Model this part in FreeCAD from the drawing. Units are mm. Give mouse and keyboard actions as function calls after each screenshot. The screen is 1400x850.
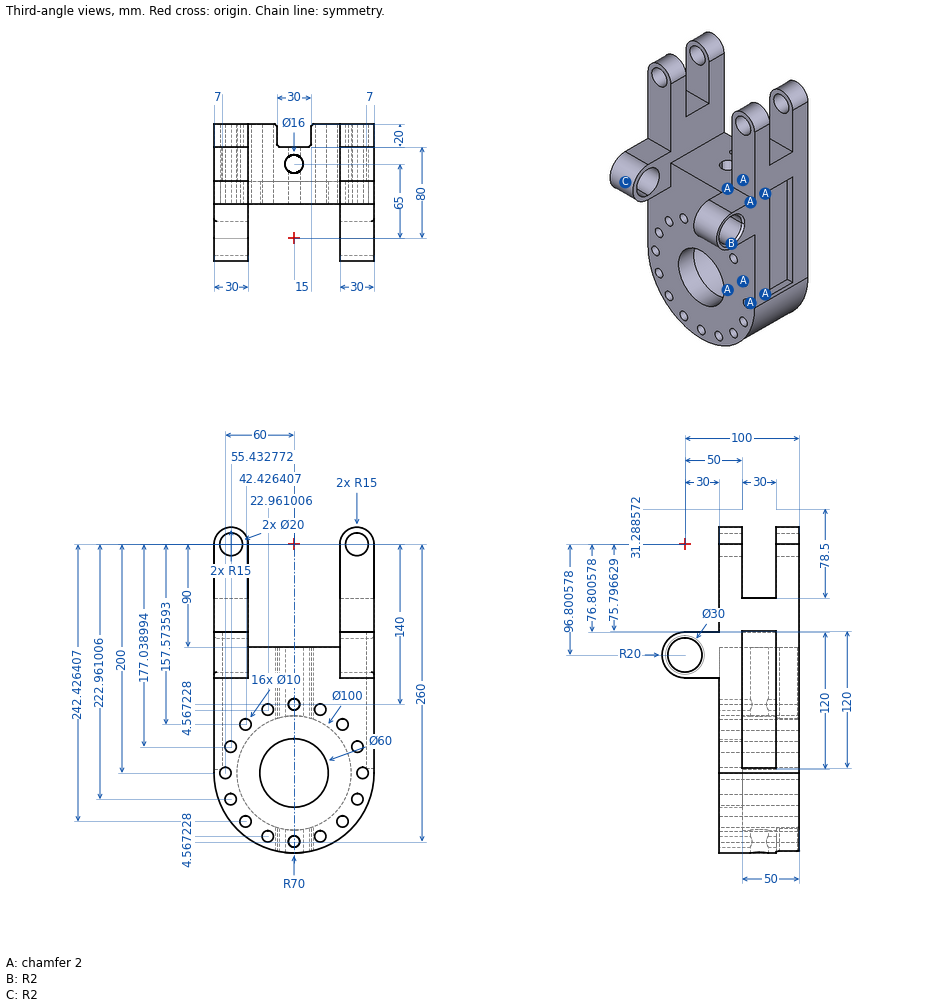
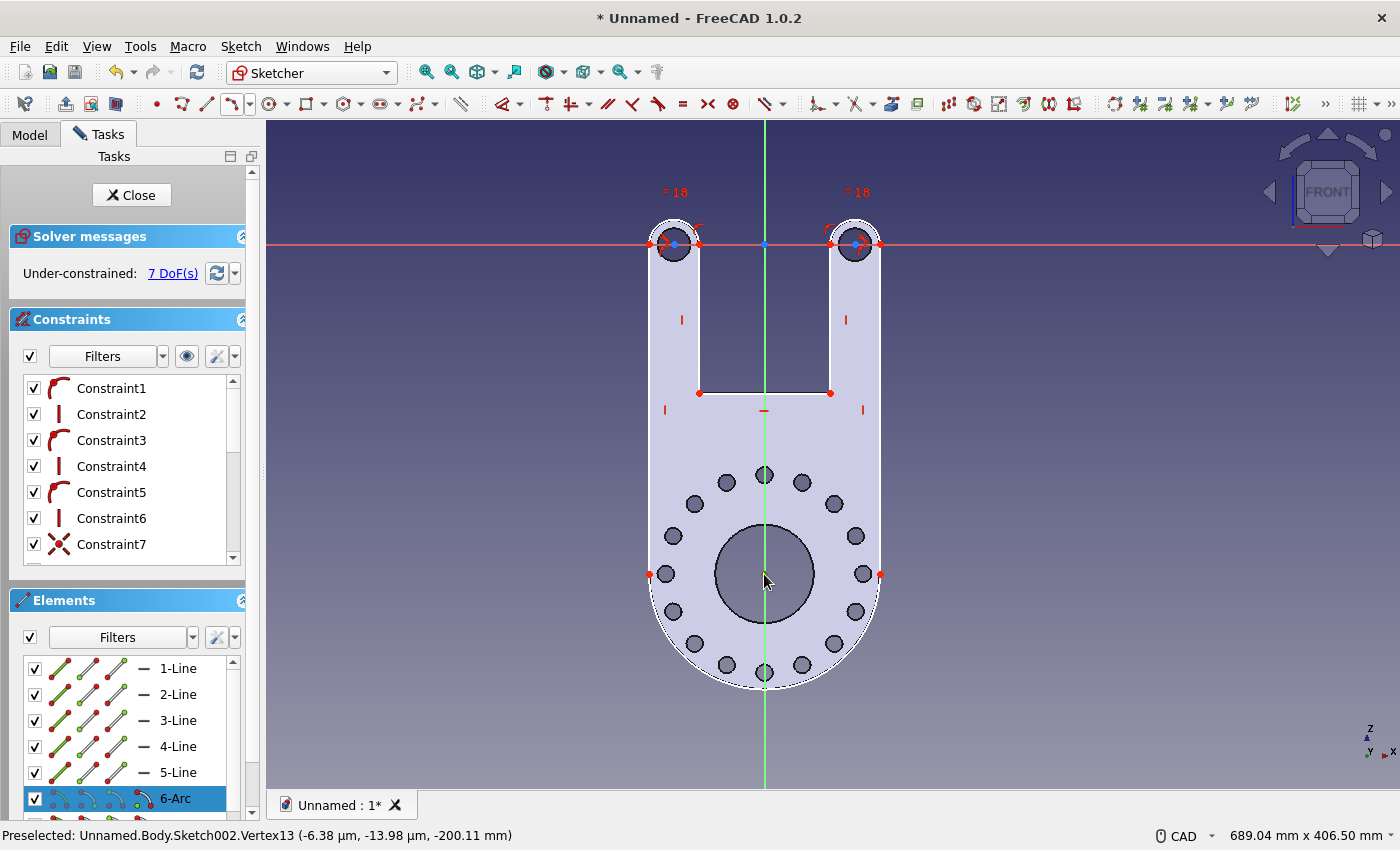
click(765, 630)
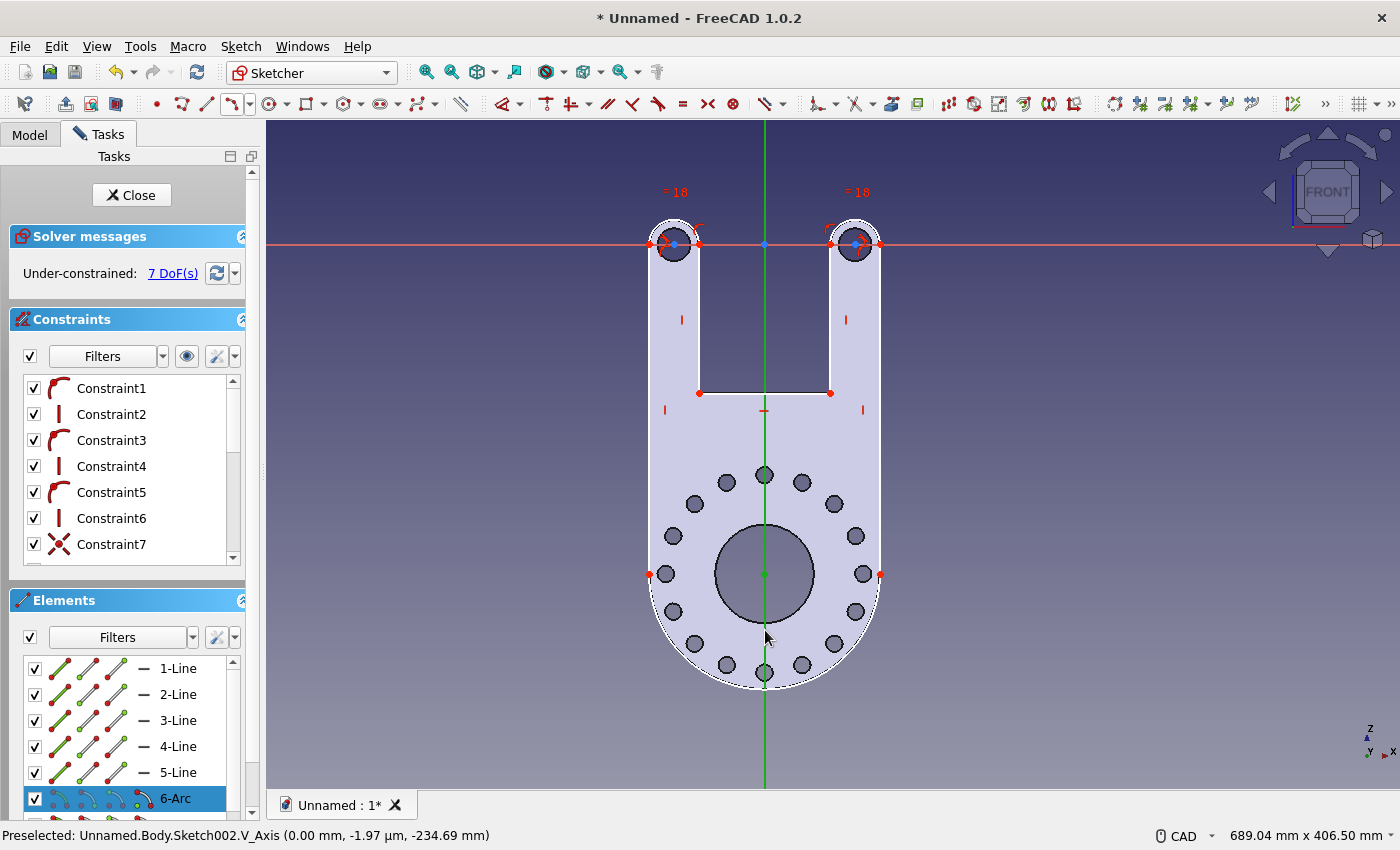
key(c)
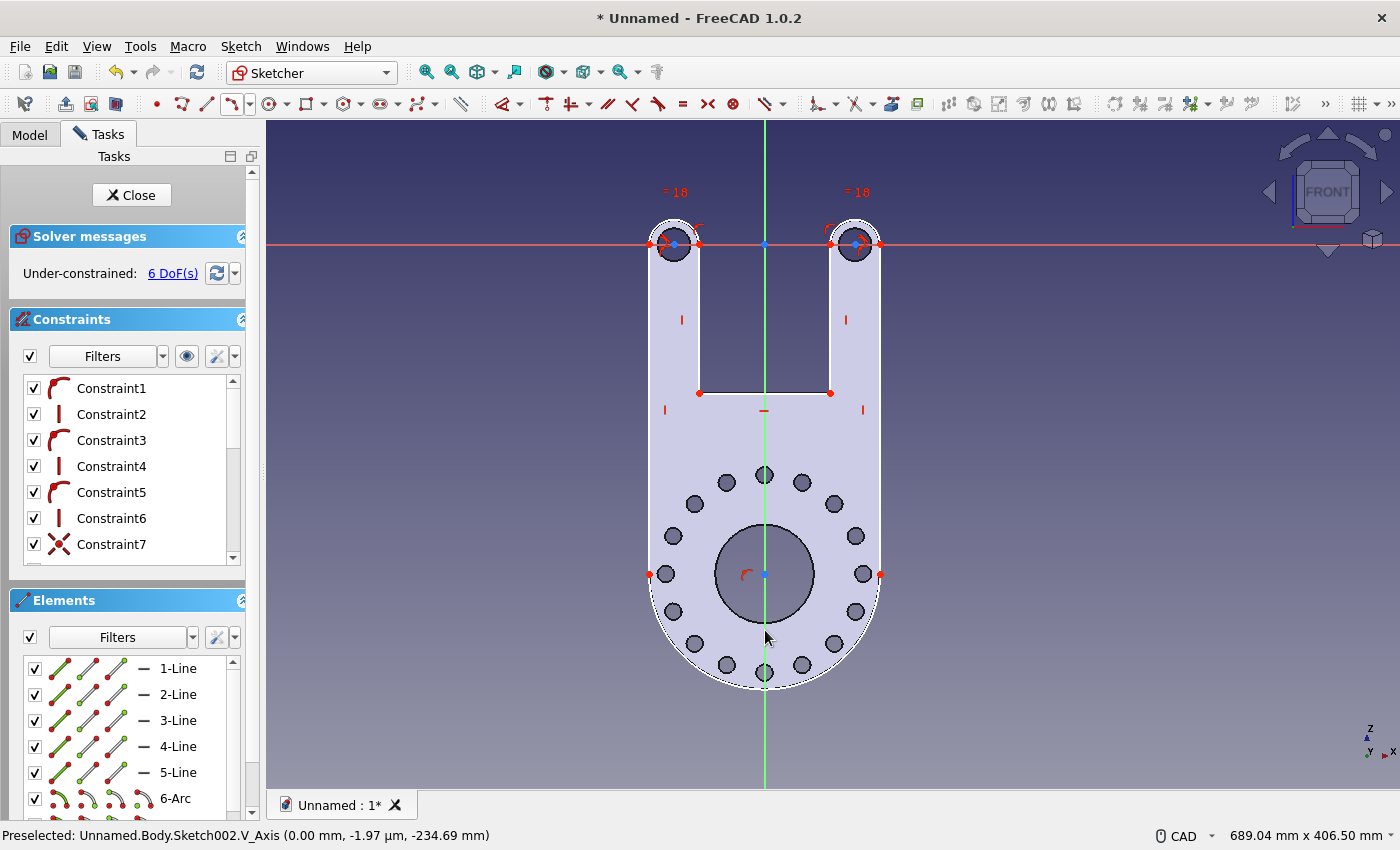
key(d)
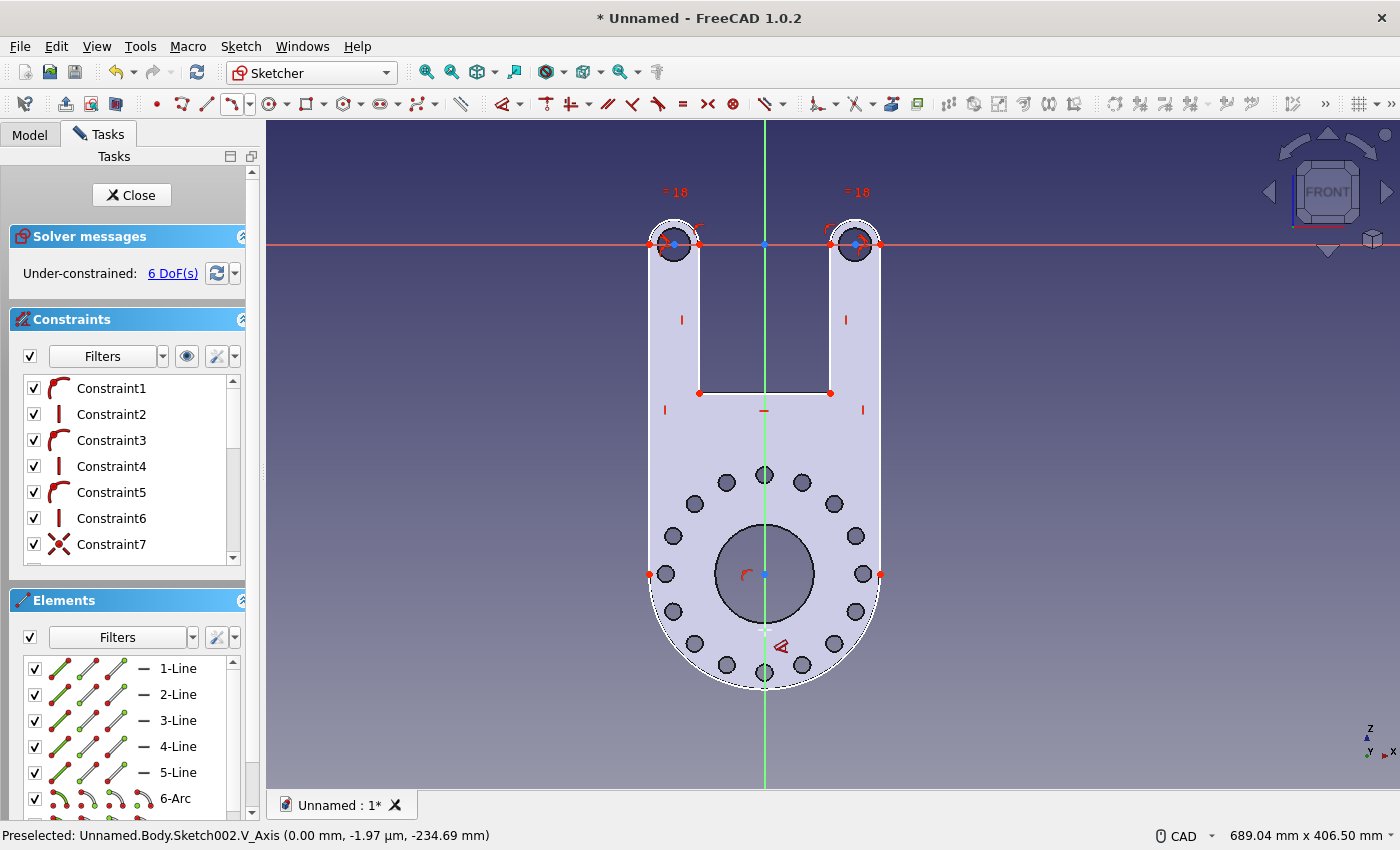
click(697, 668)
click(678, 694)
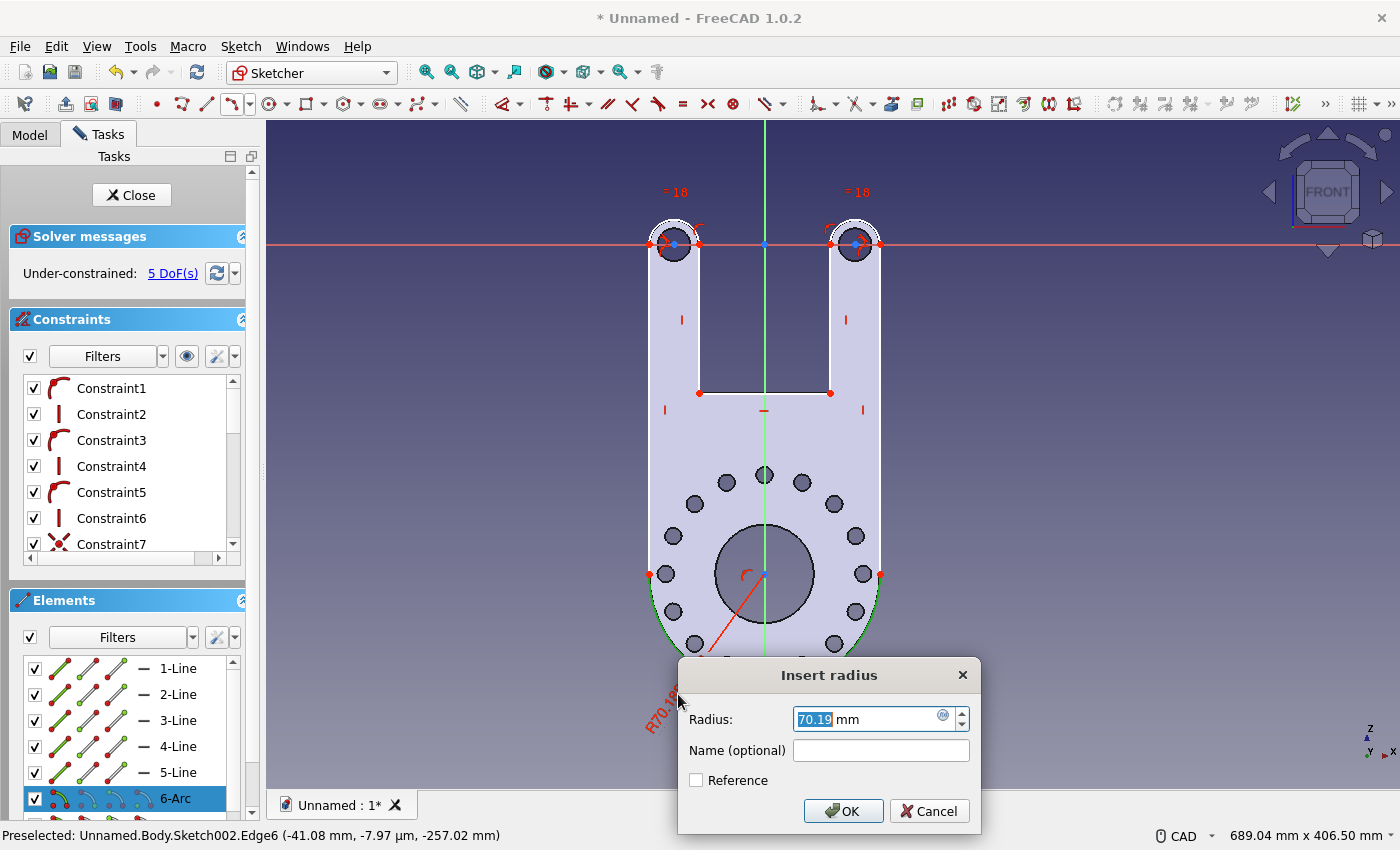
text(70)
key(Return)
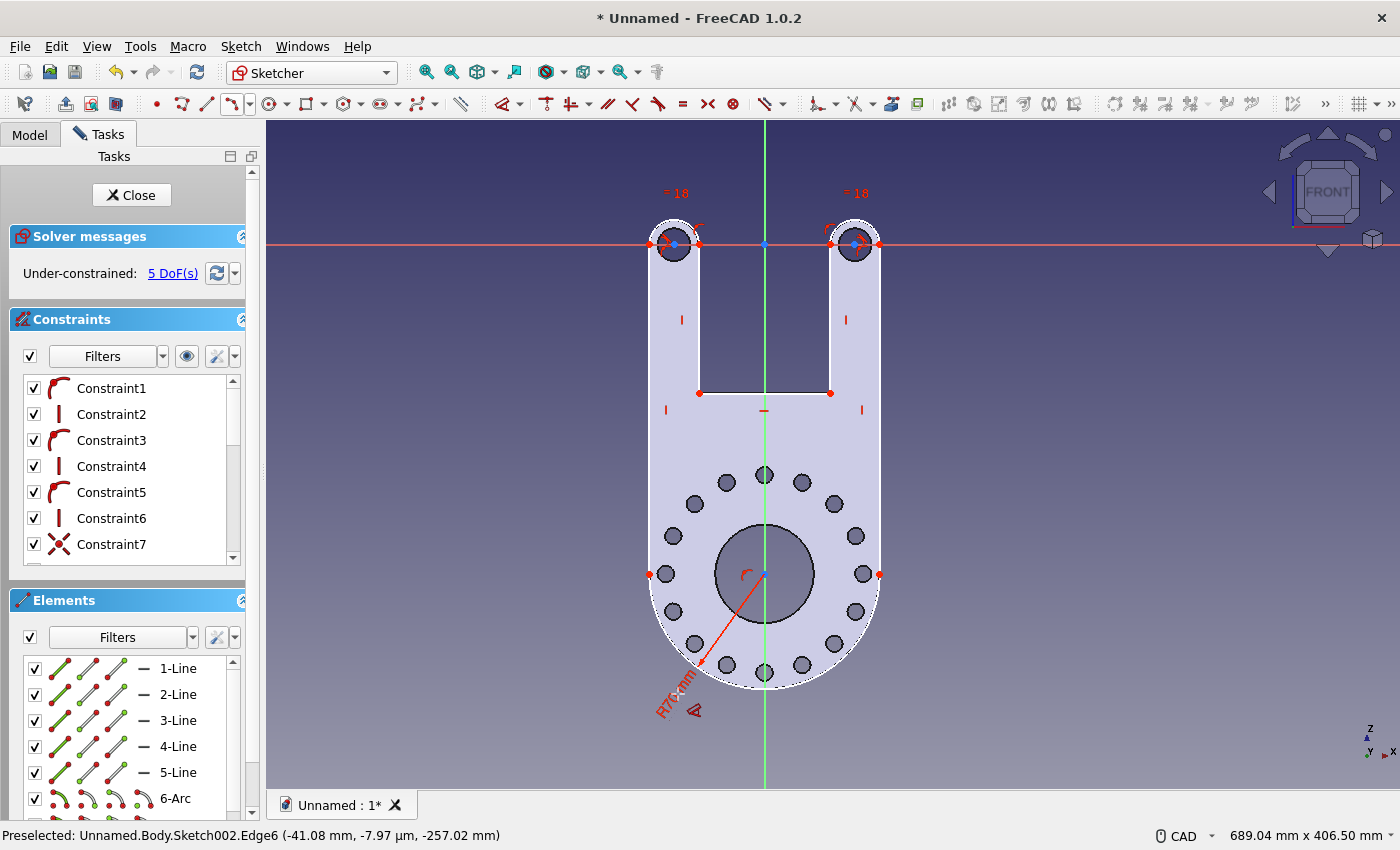
scroll(869, 225, up, 3)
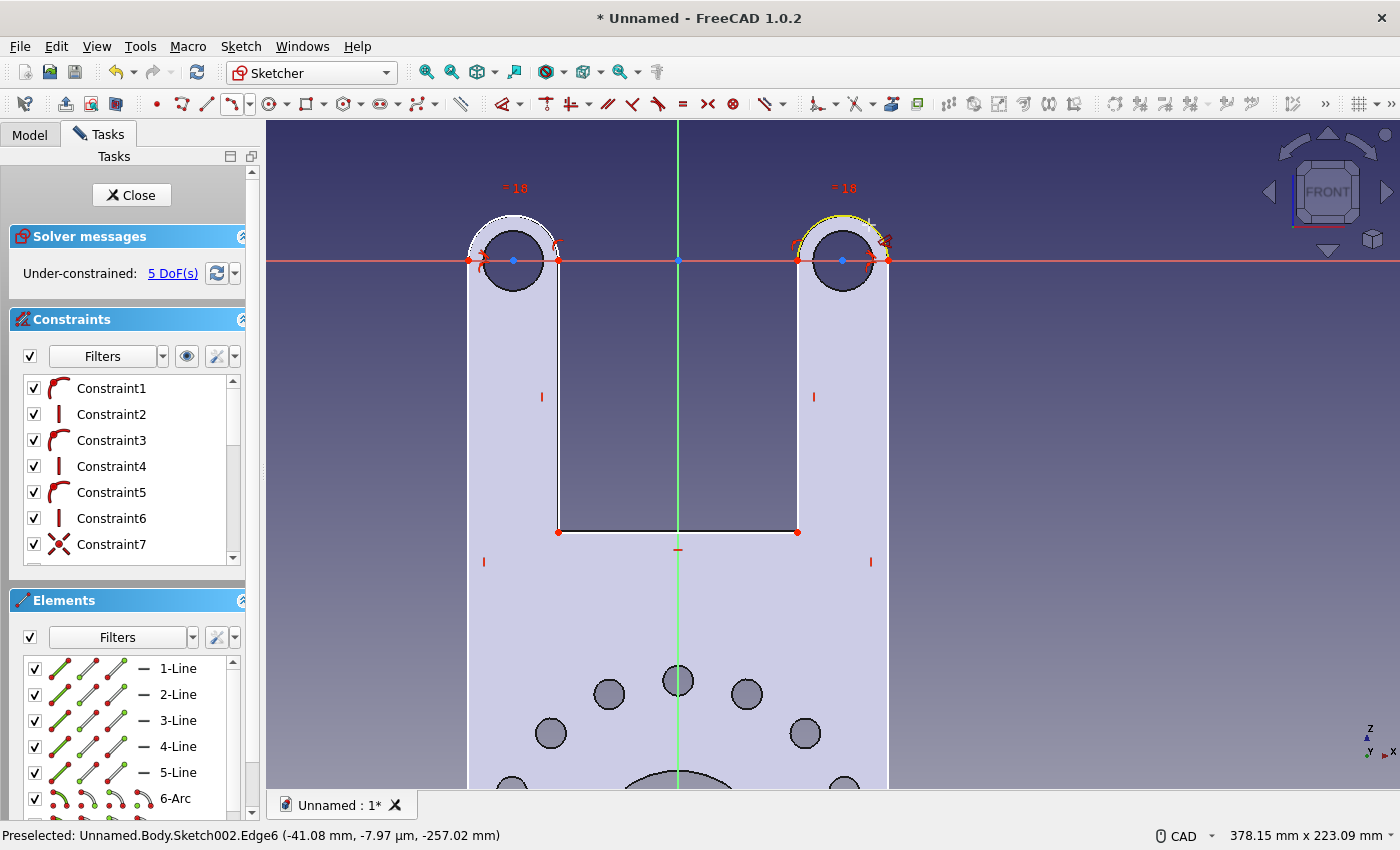
click(869, 224)
click(888, 198)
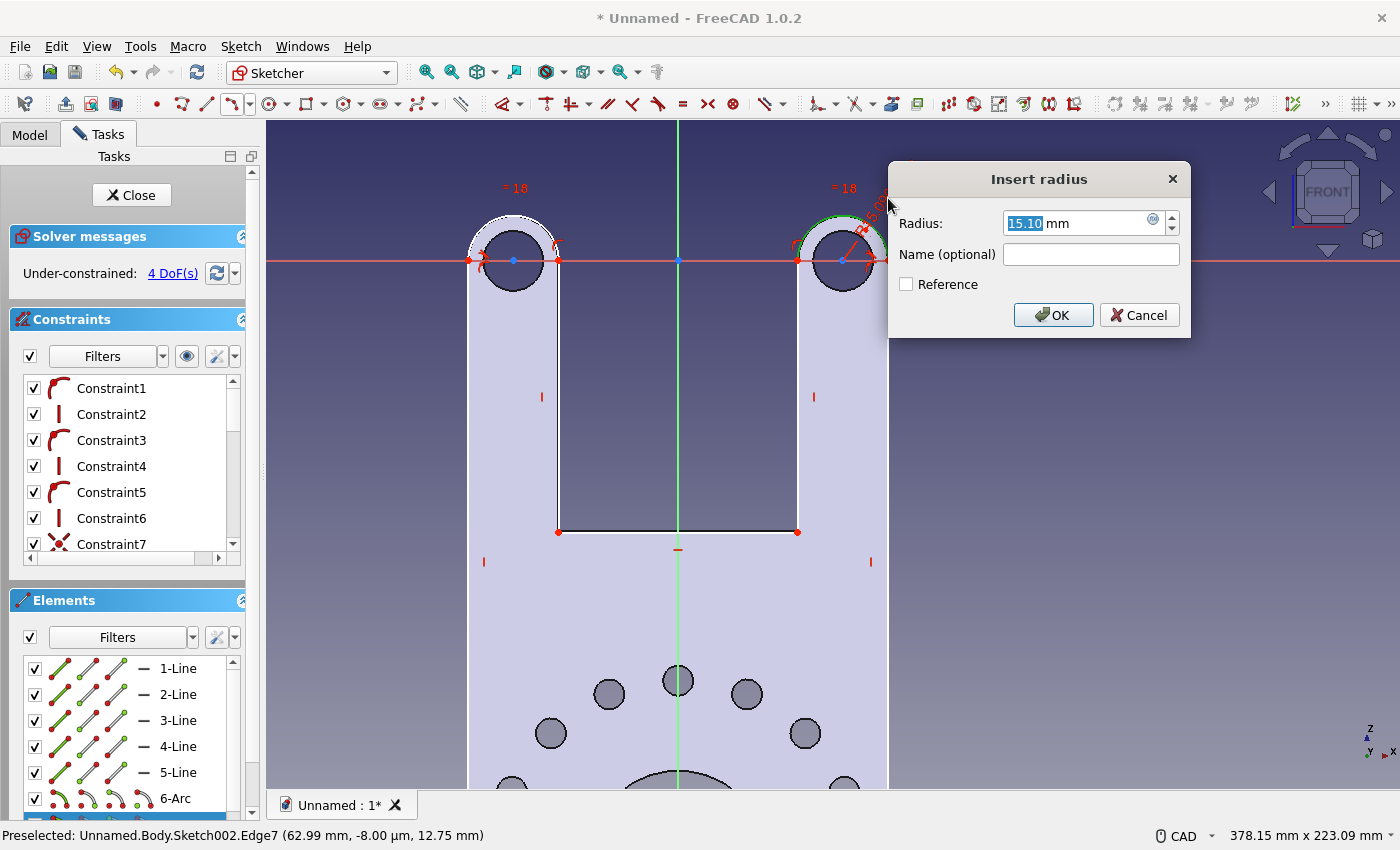
text(15)
key(Return)